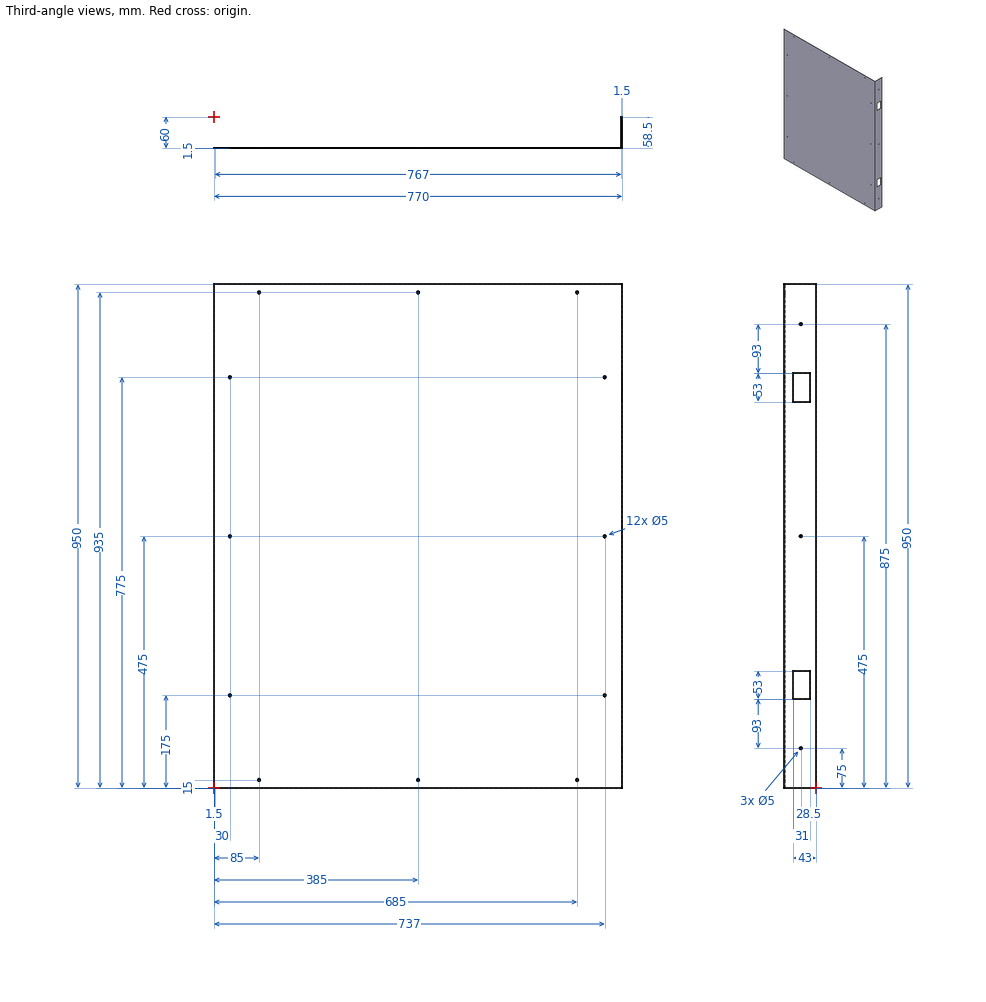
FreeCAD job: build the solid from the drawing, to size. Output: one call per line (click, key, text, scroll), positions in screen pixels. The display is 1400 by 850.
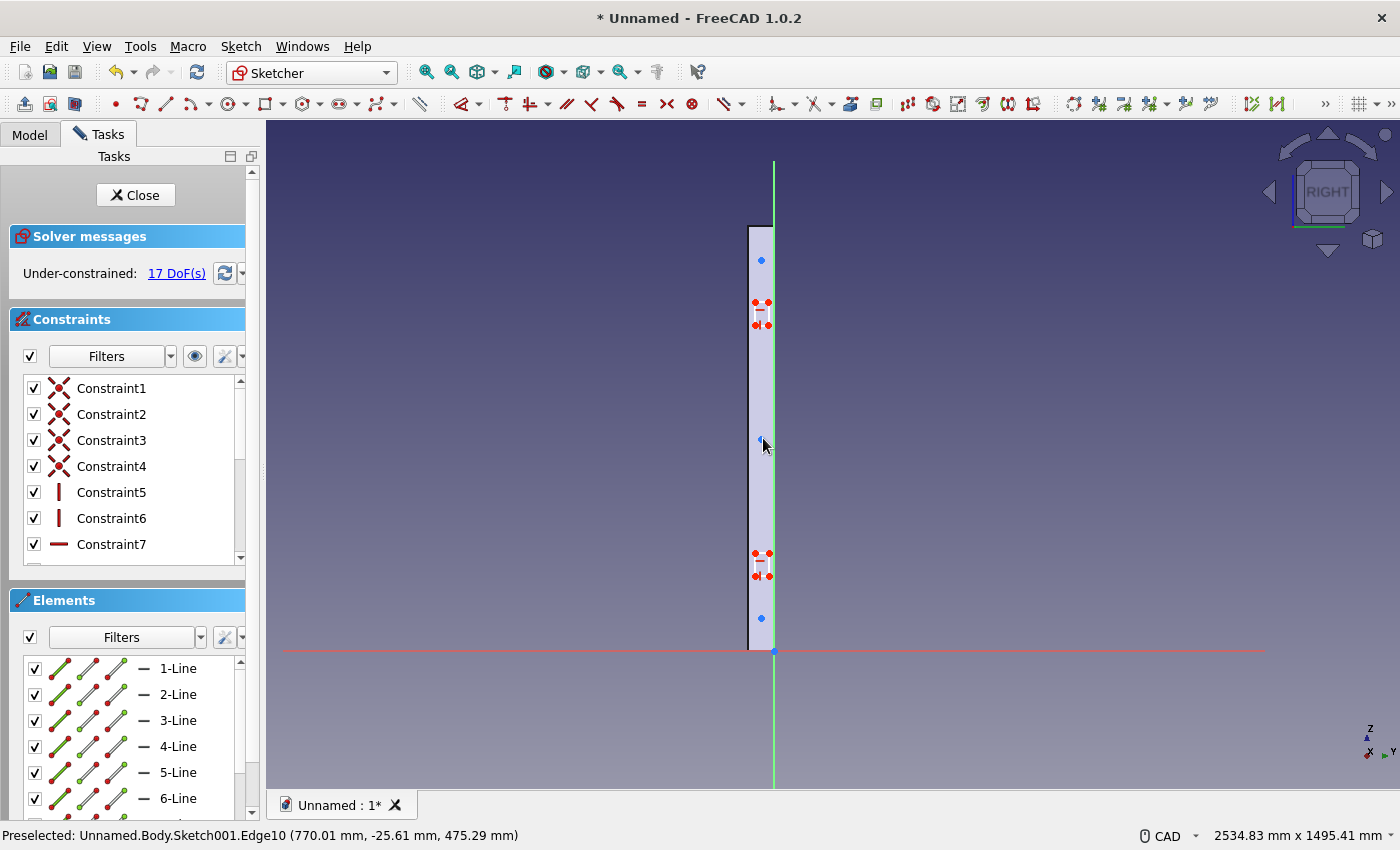
scroll(763, 259, up, 10)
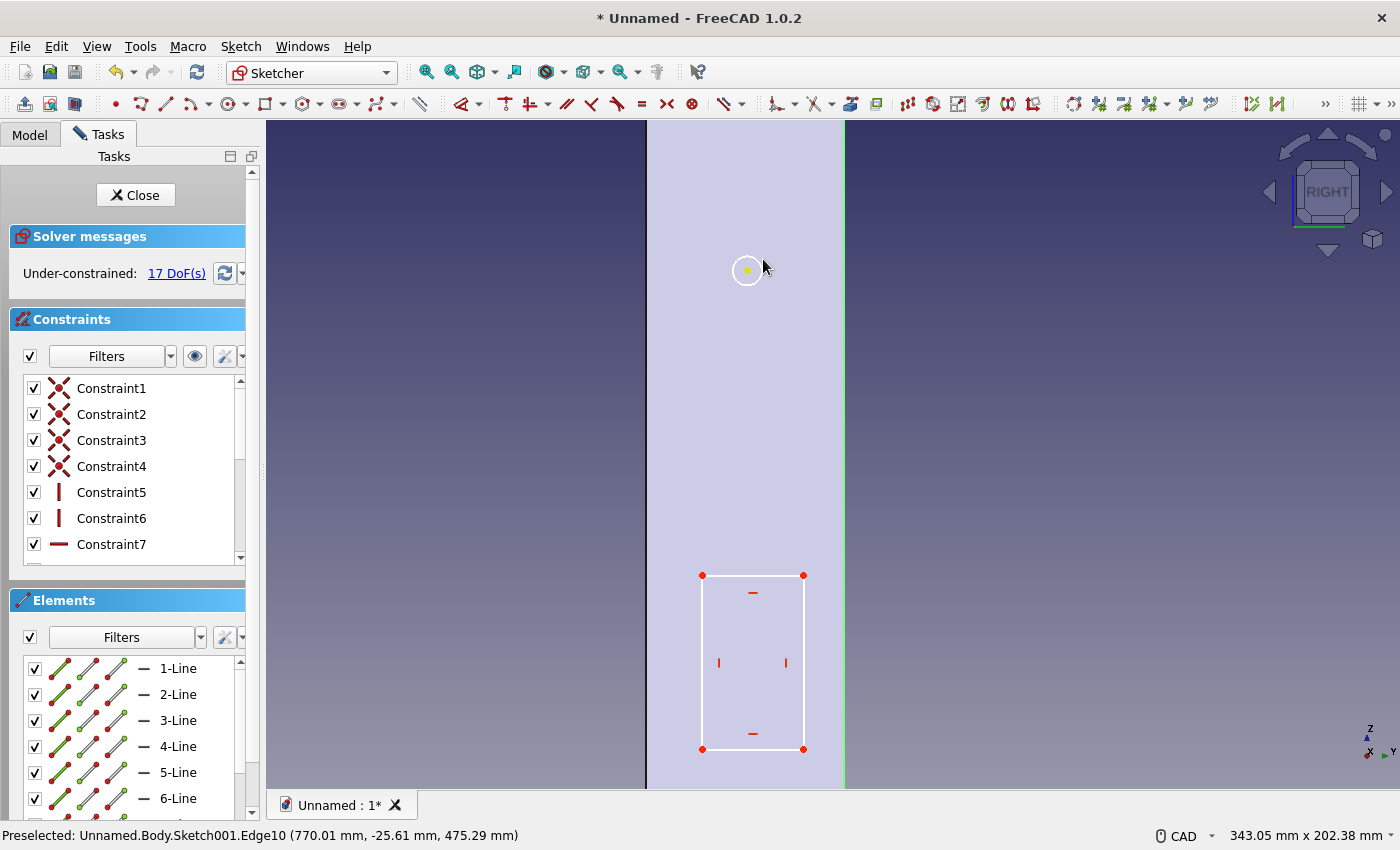
click(758, 261)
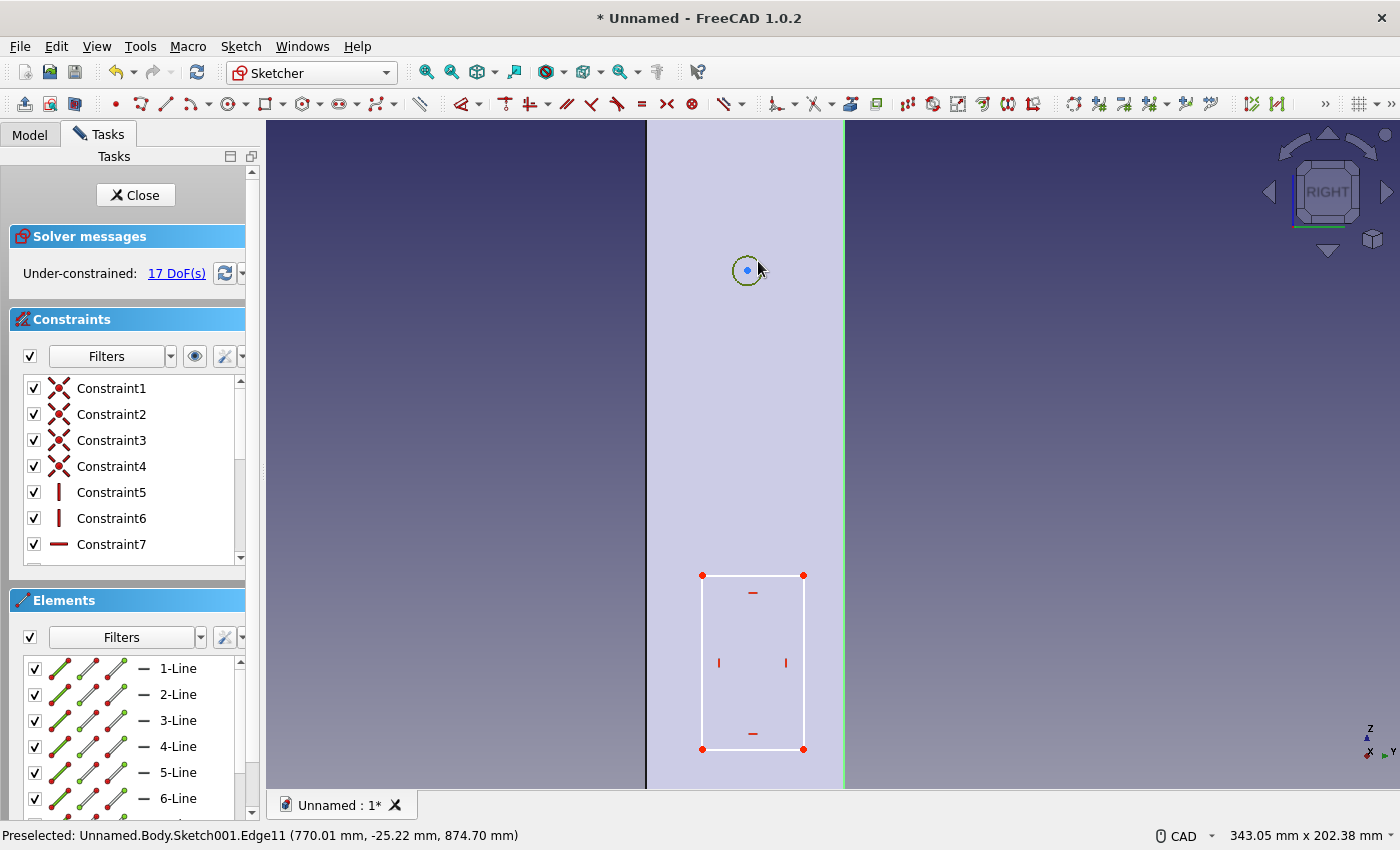
click(642, 104)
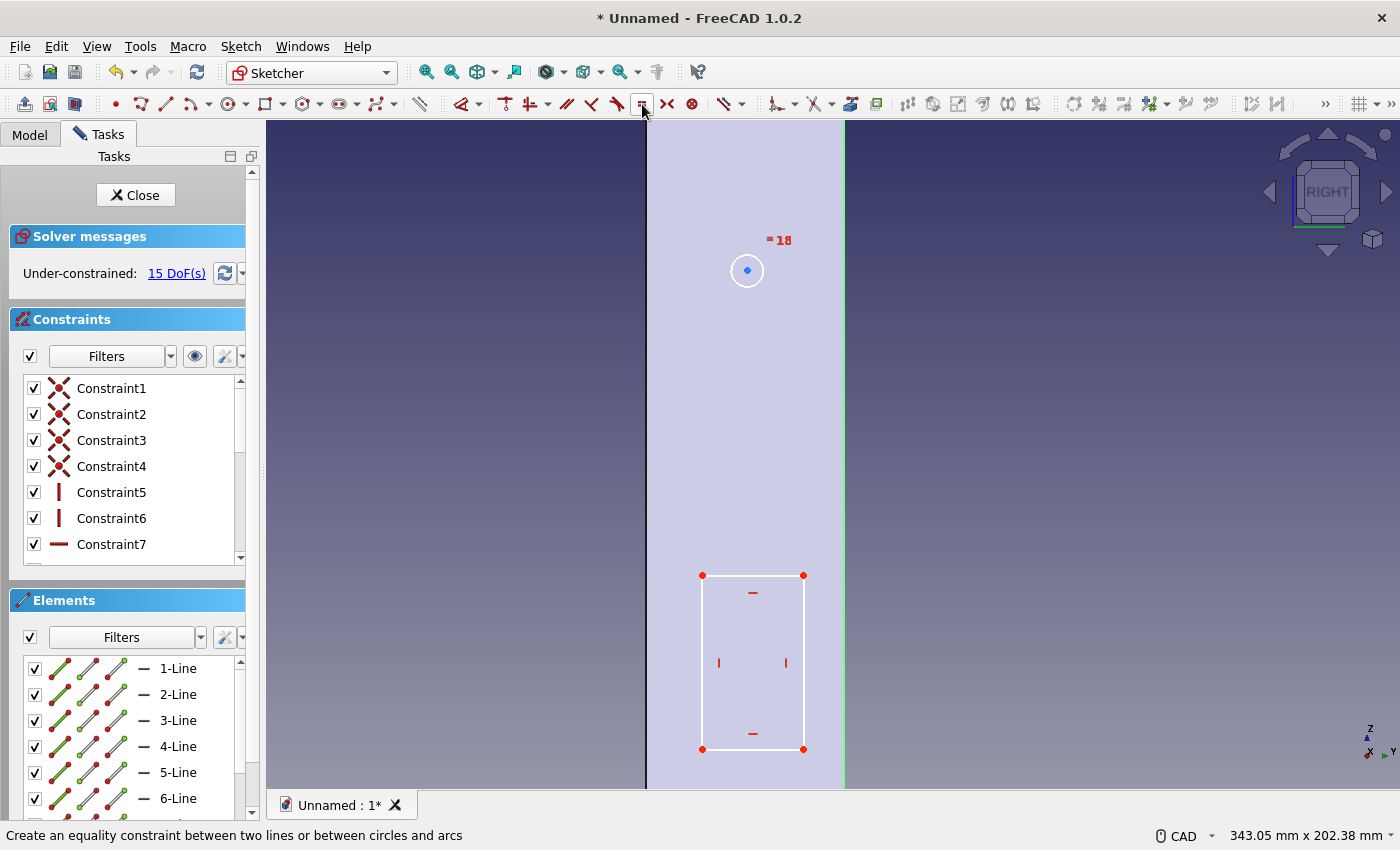
key(d)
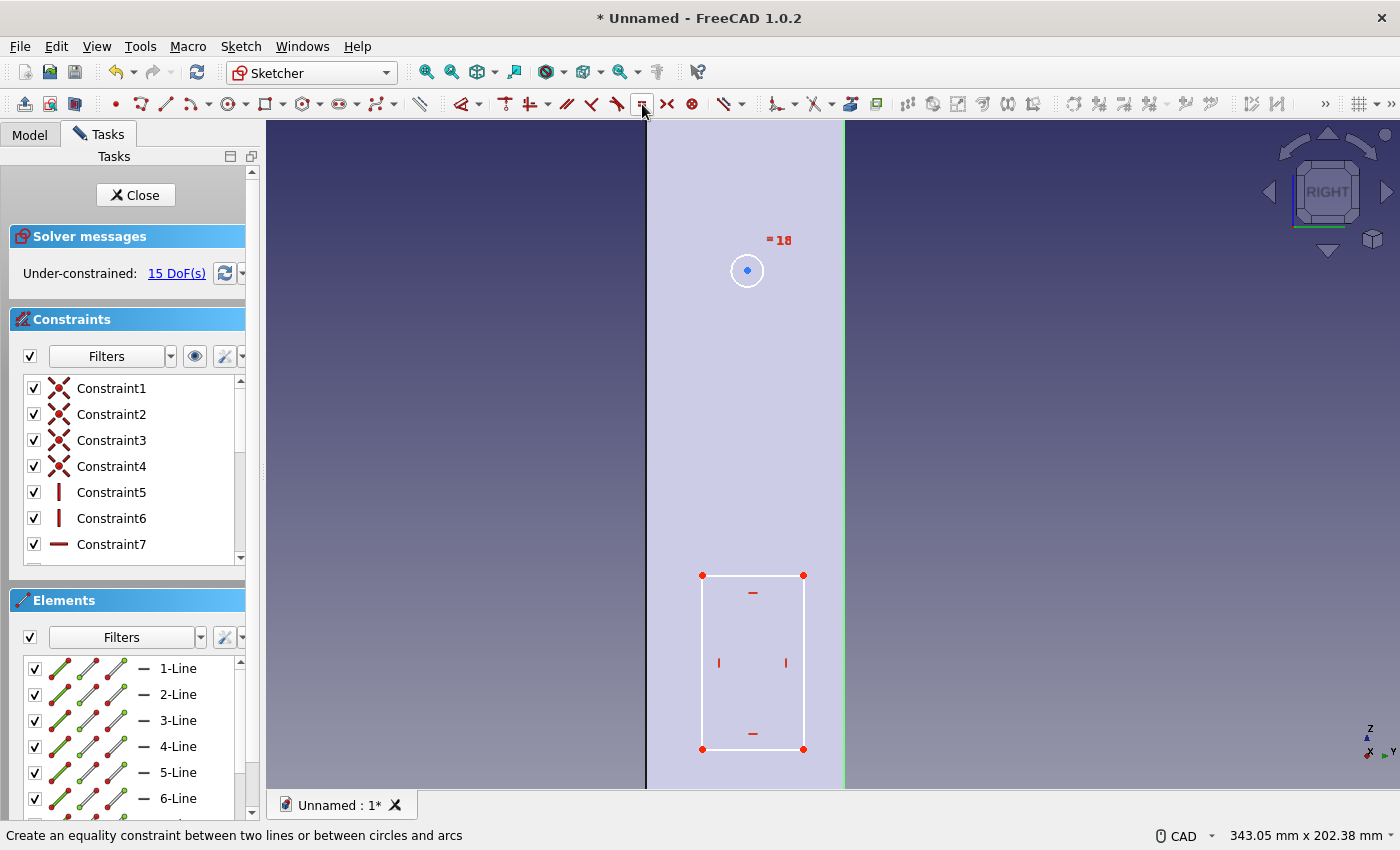
scroll(763, 259, down, 10)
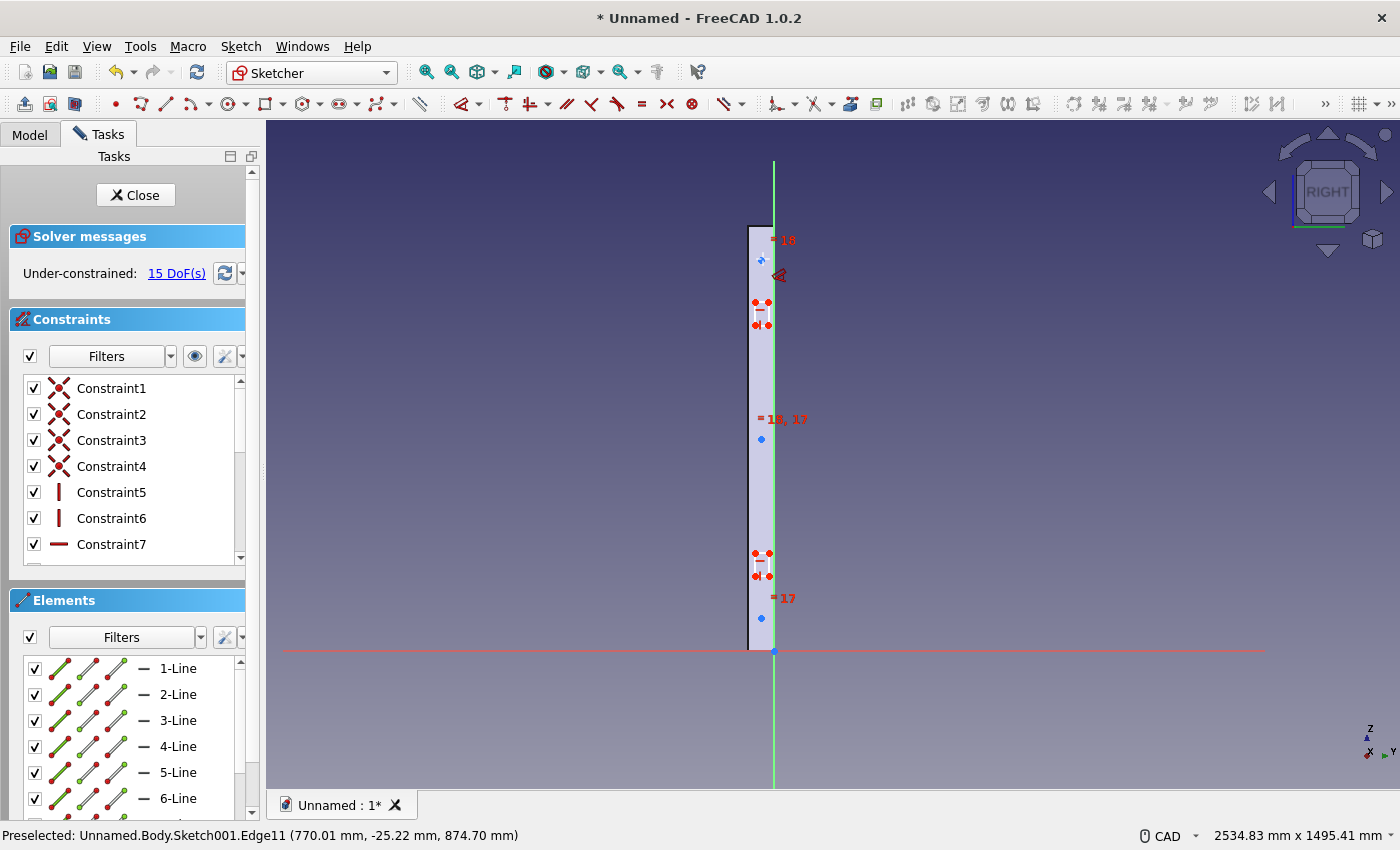
scroll(763, 617, up, 15)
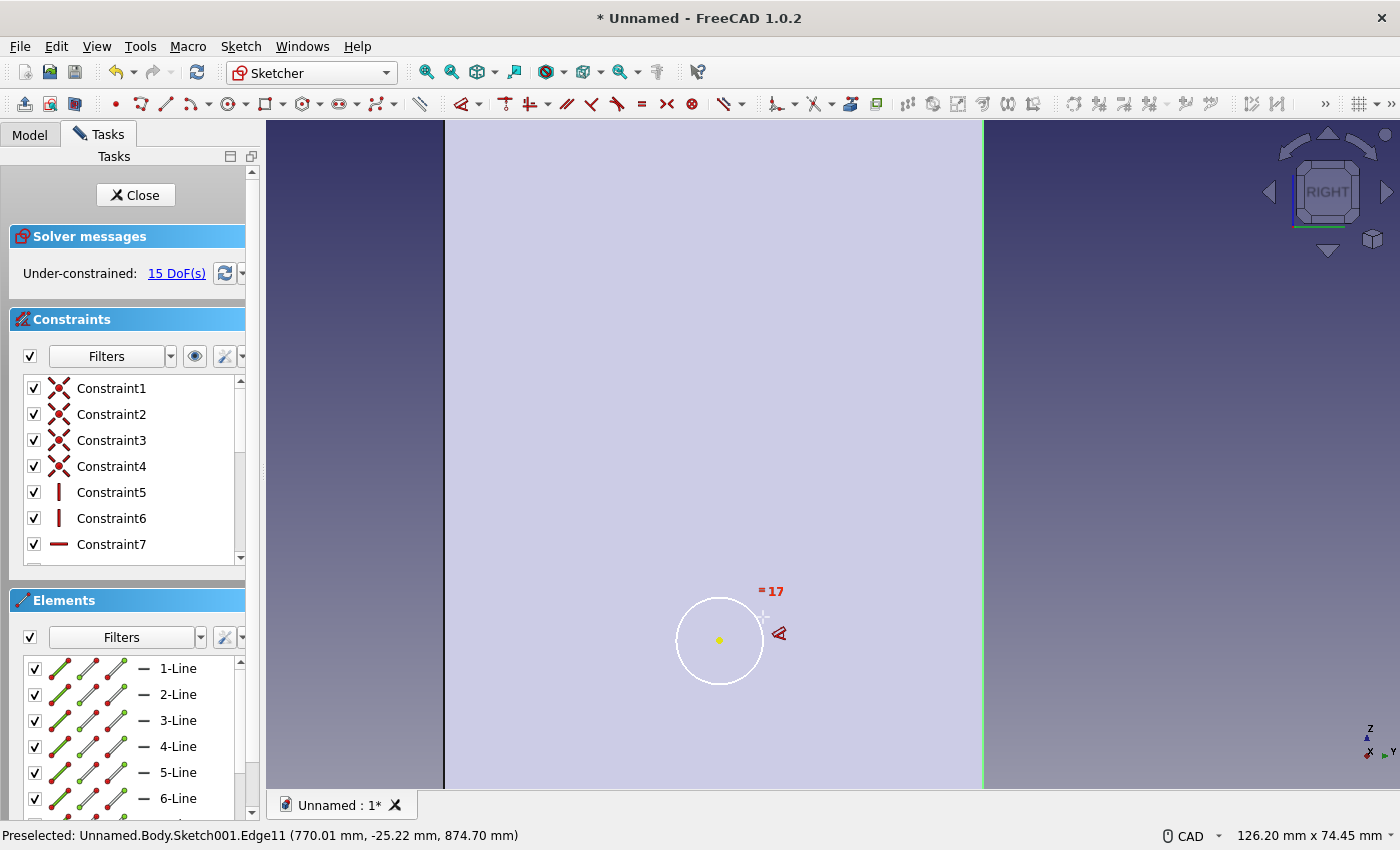
click(750, 610)
click(772, 587)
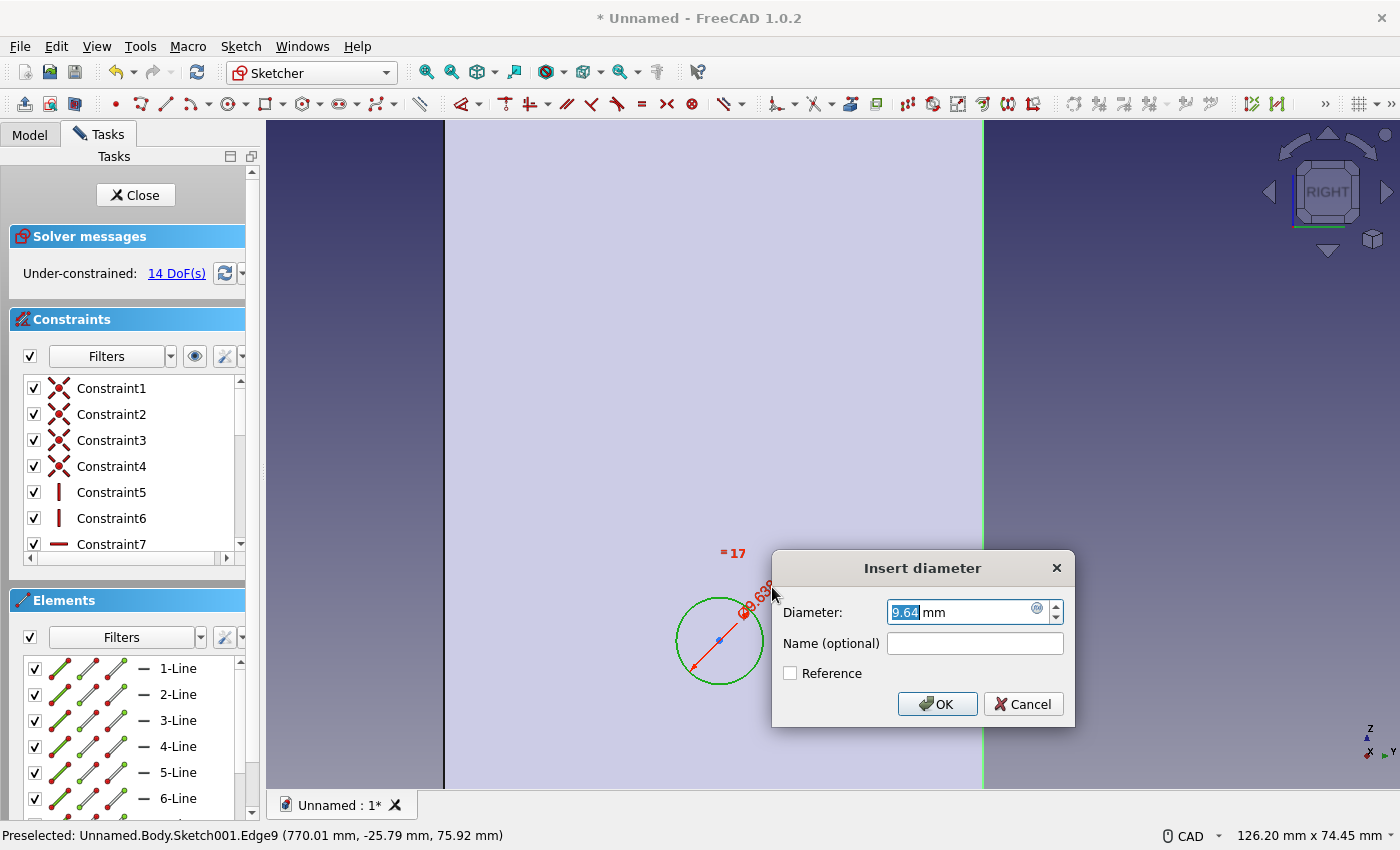
text(5)
key(Return)